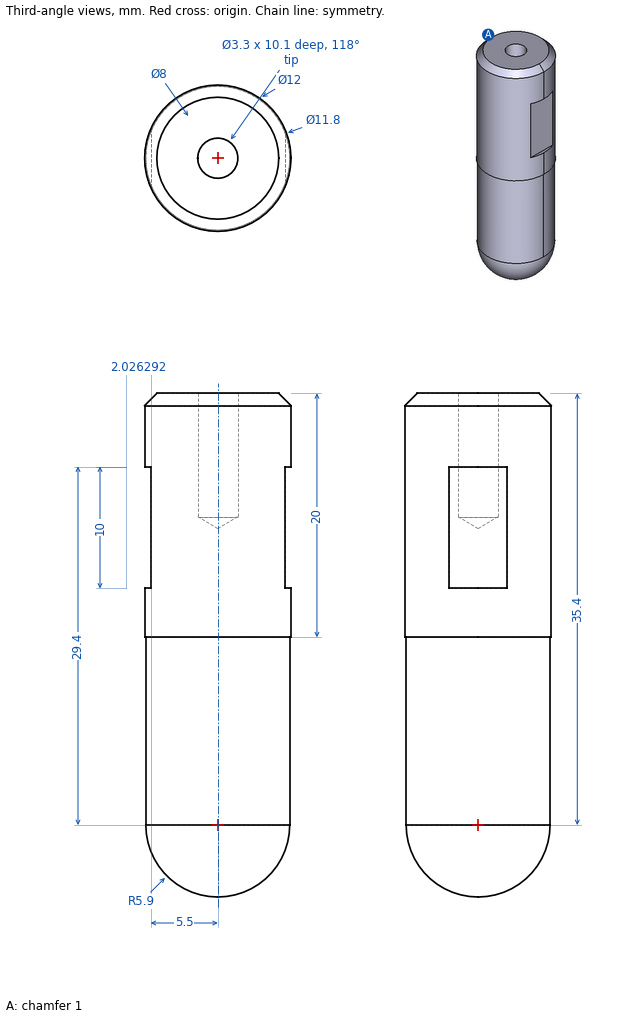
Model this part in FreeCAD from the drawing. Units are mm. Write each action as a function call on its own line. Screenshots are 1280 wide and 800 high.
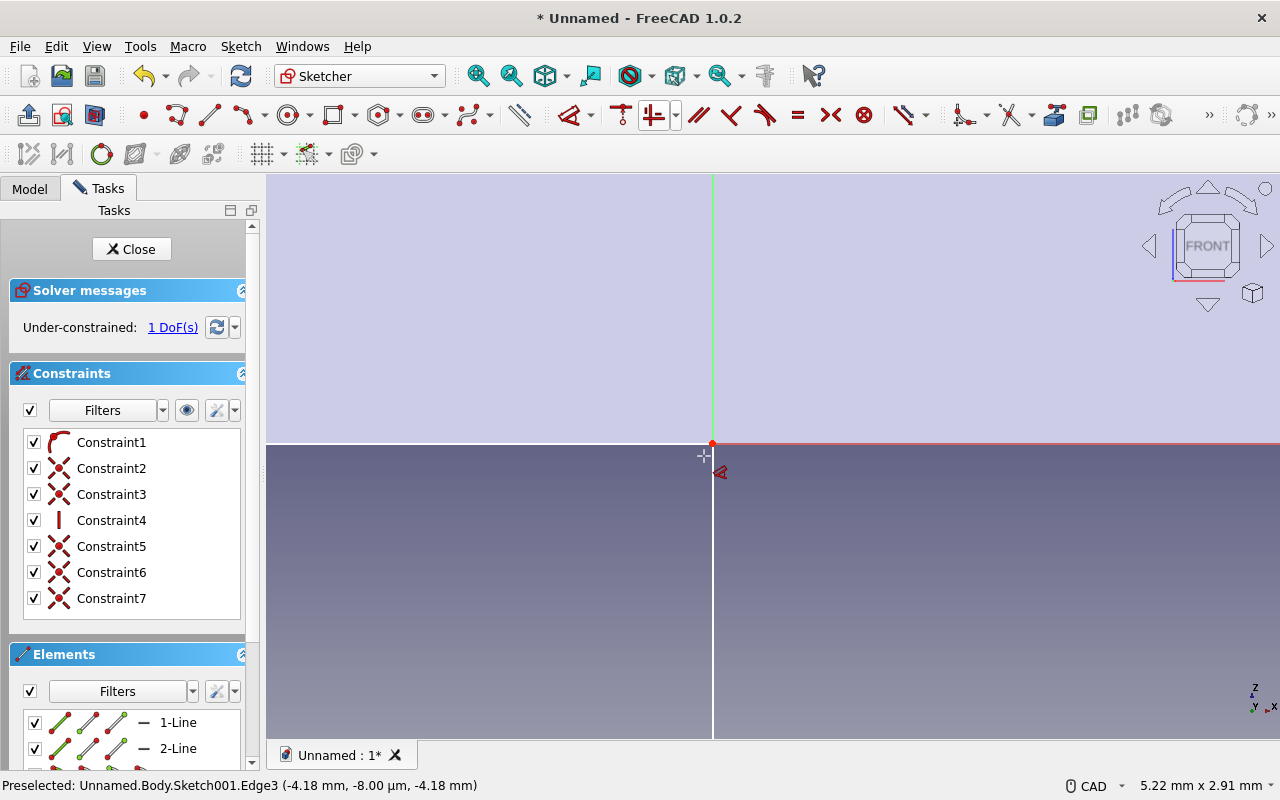
scroll(948, 215, down, 6)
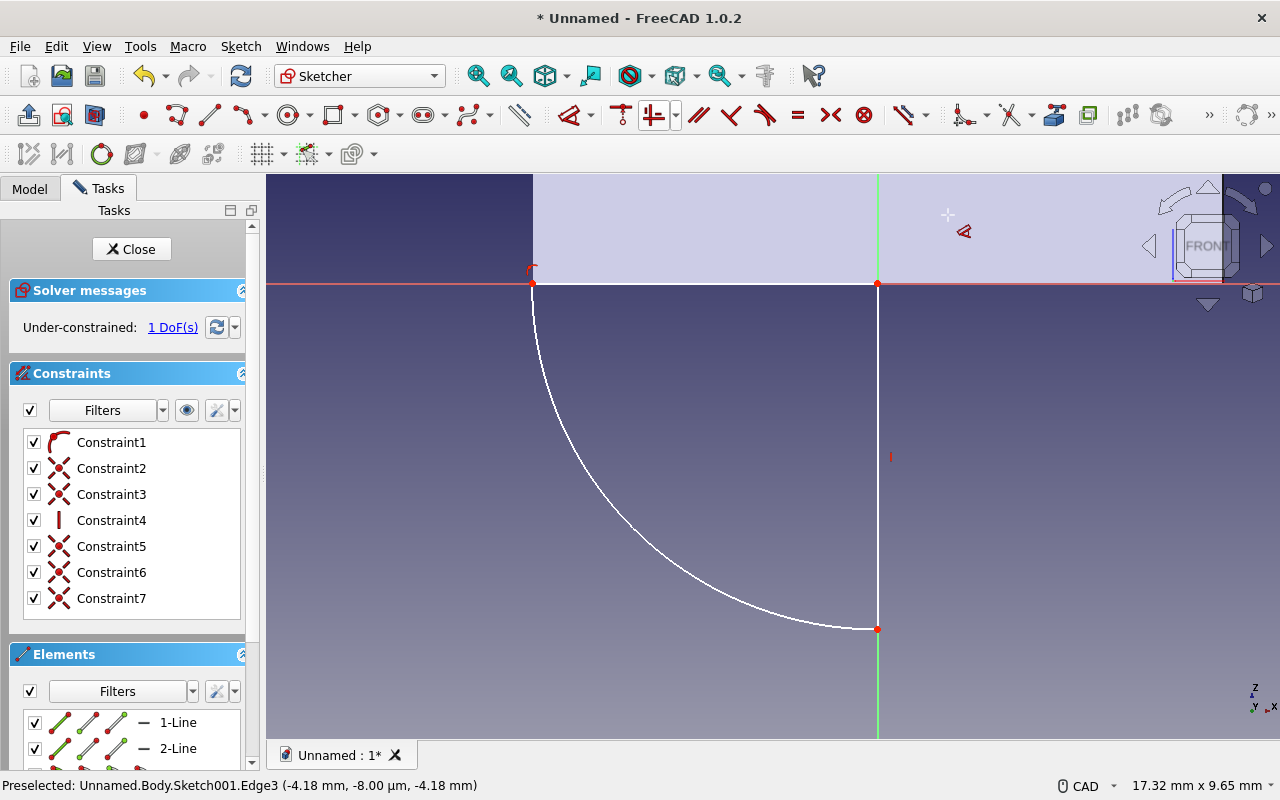
click(570, 441)
click(542, 456)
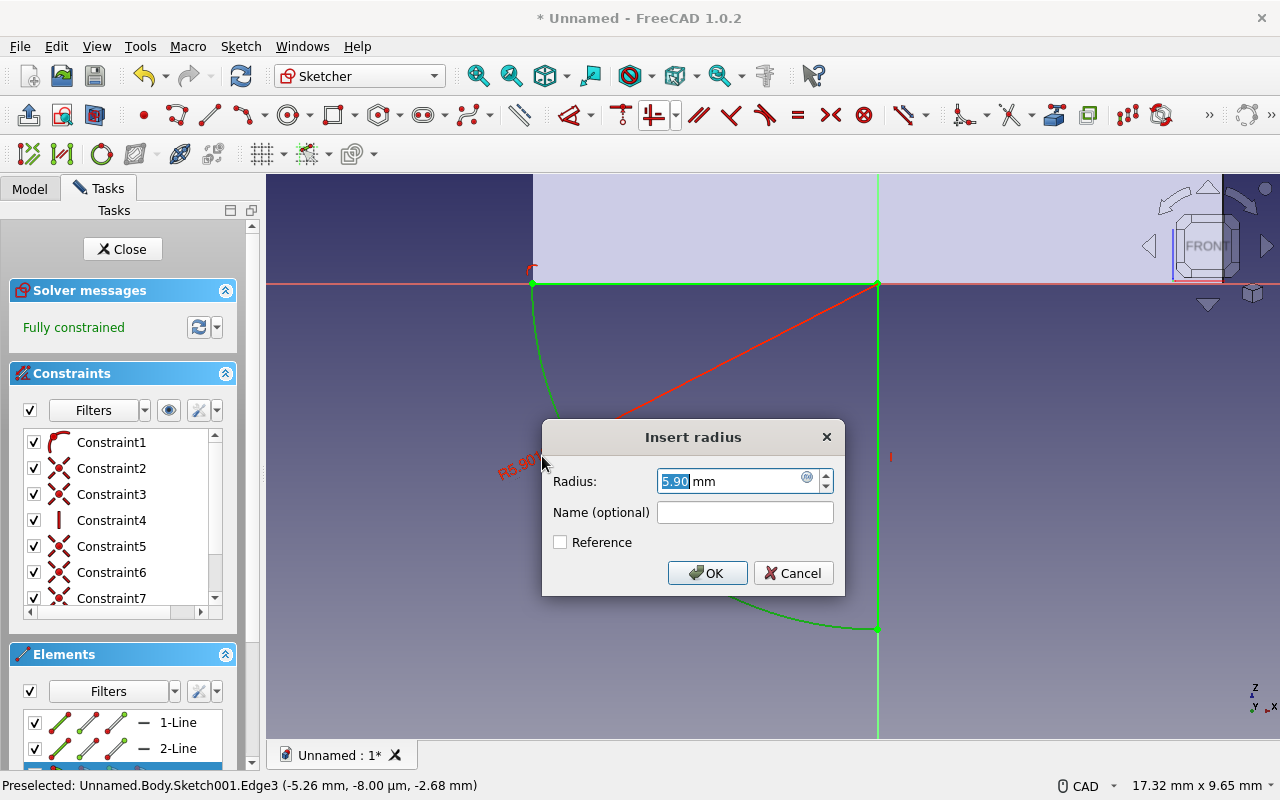
text(5.9)
key(Return)
key(Escape)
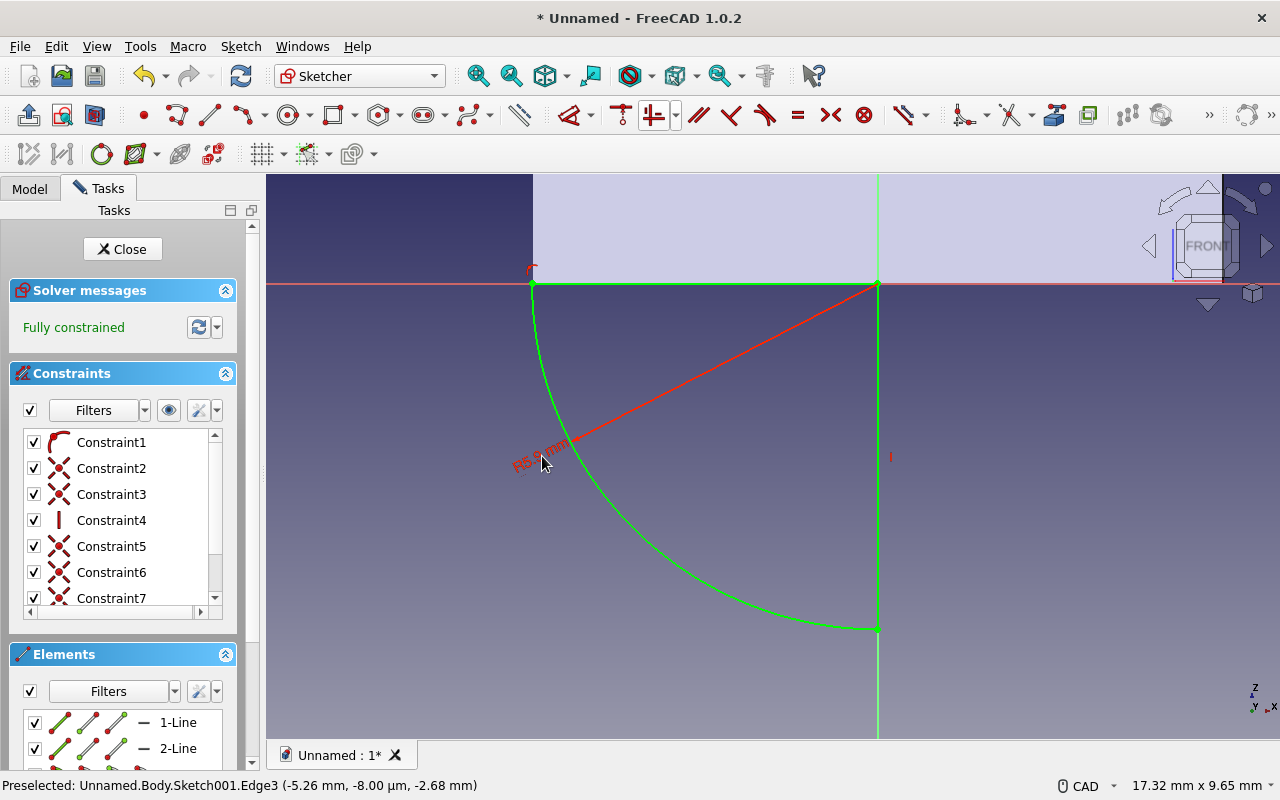
click(123, 249)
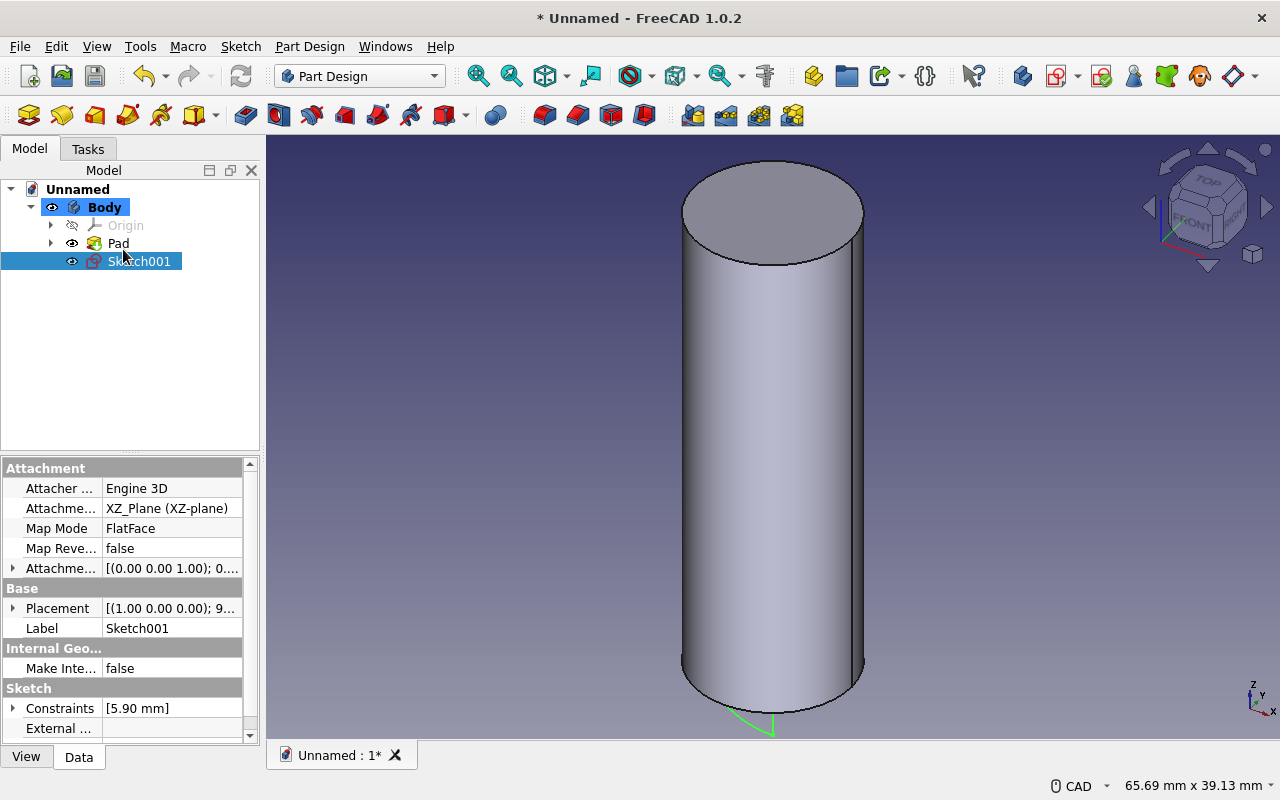
click(62, 116)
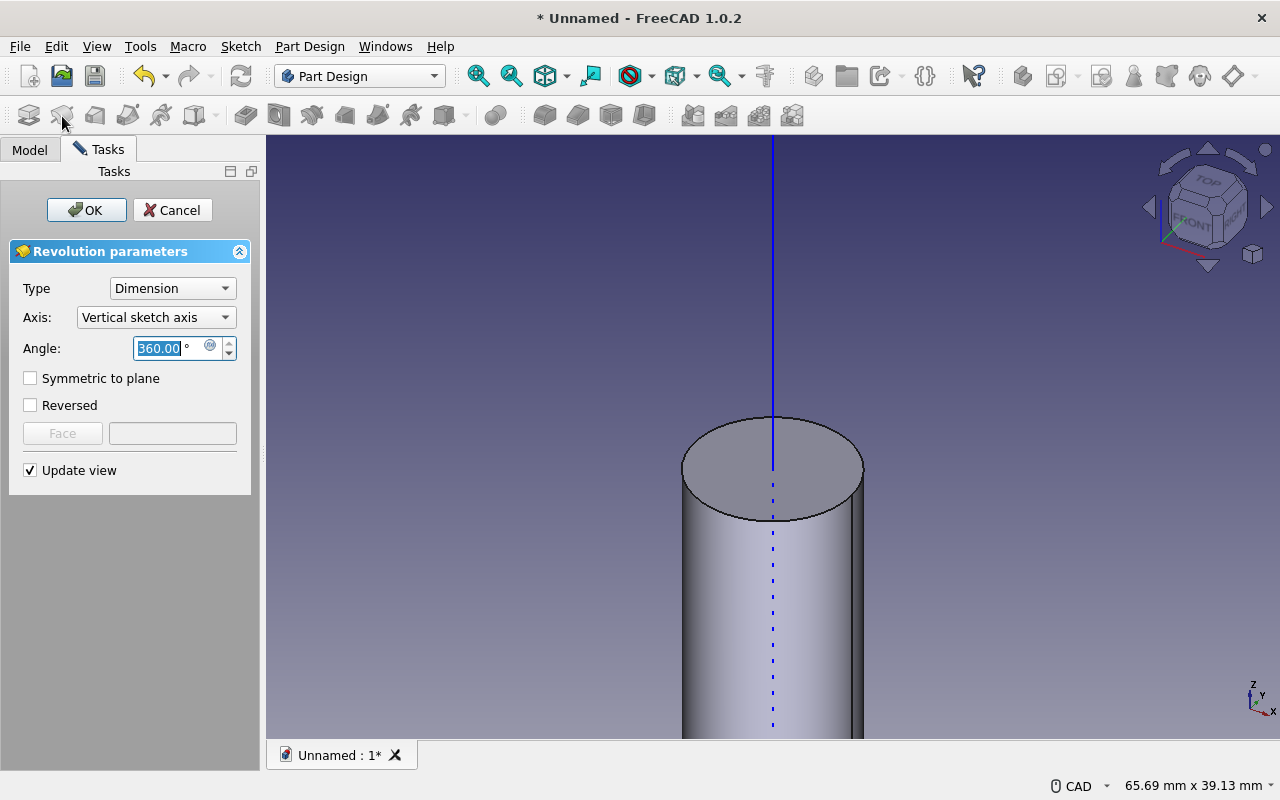
click(87, 210)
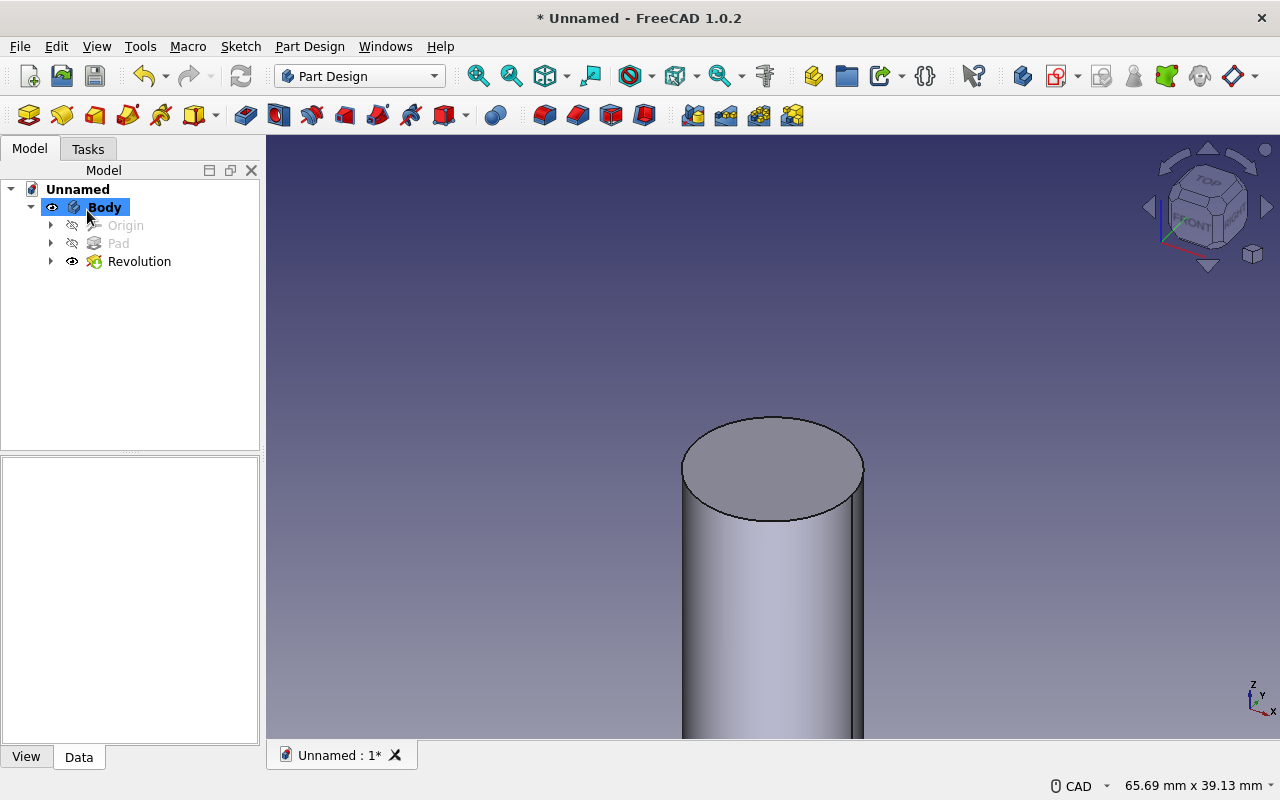
click(479, 76)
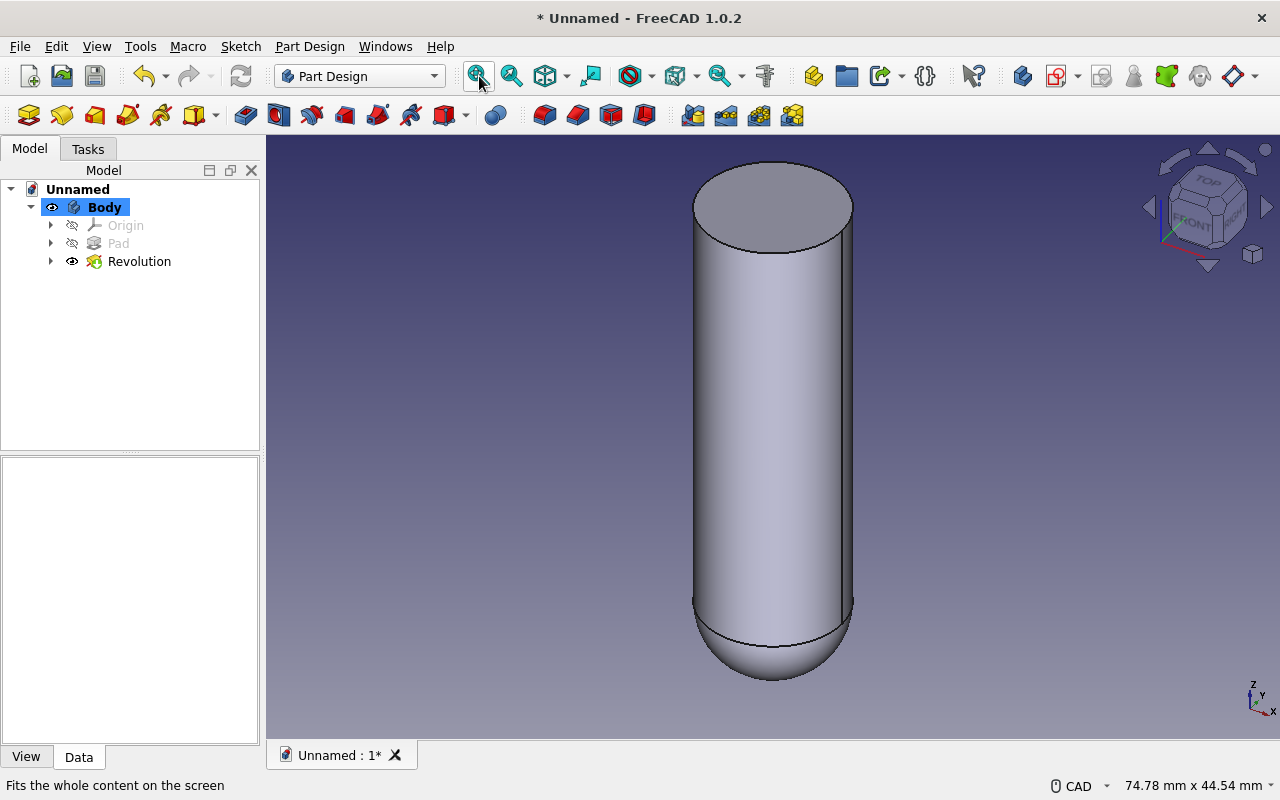
click(773, 207)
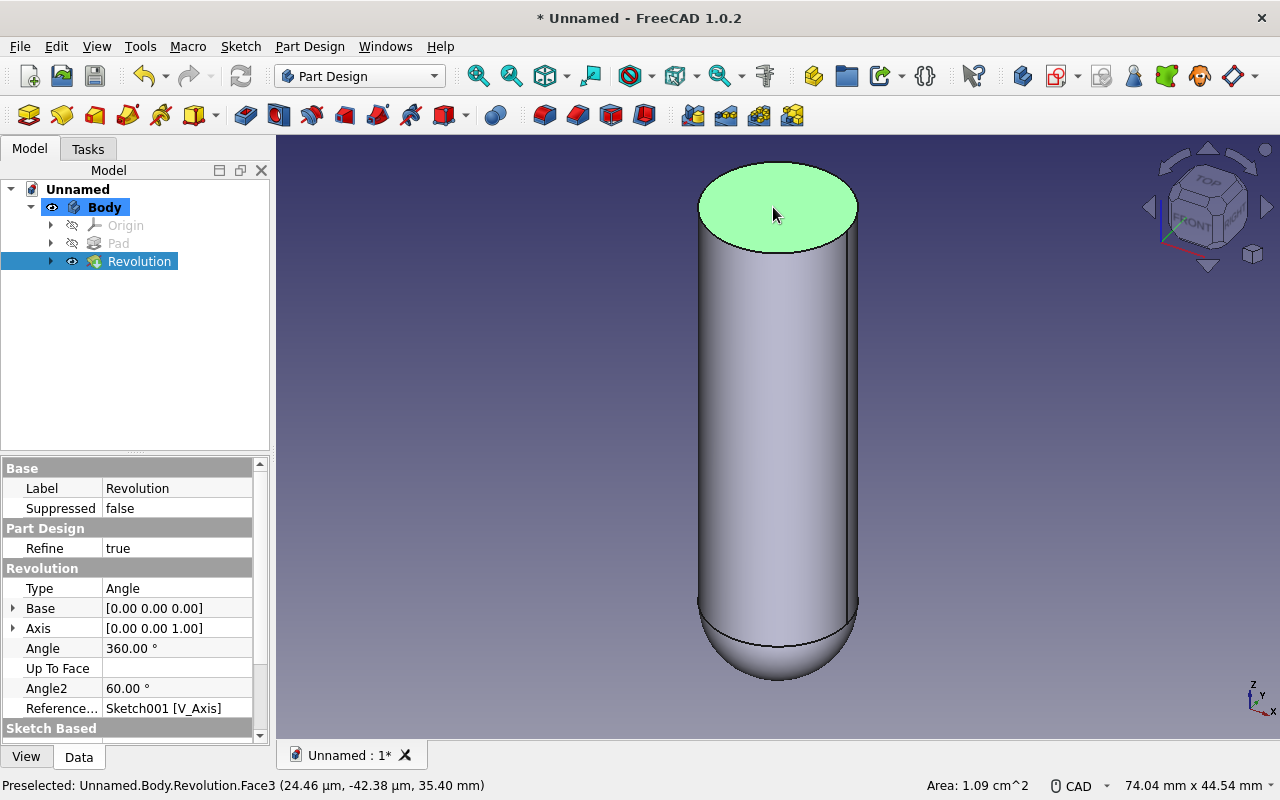
click(1056, 76)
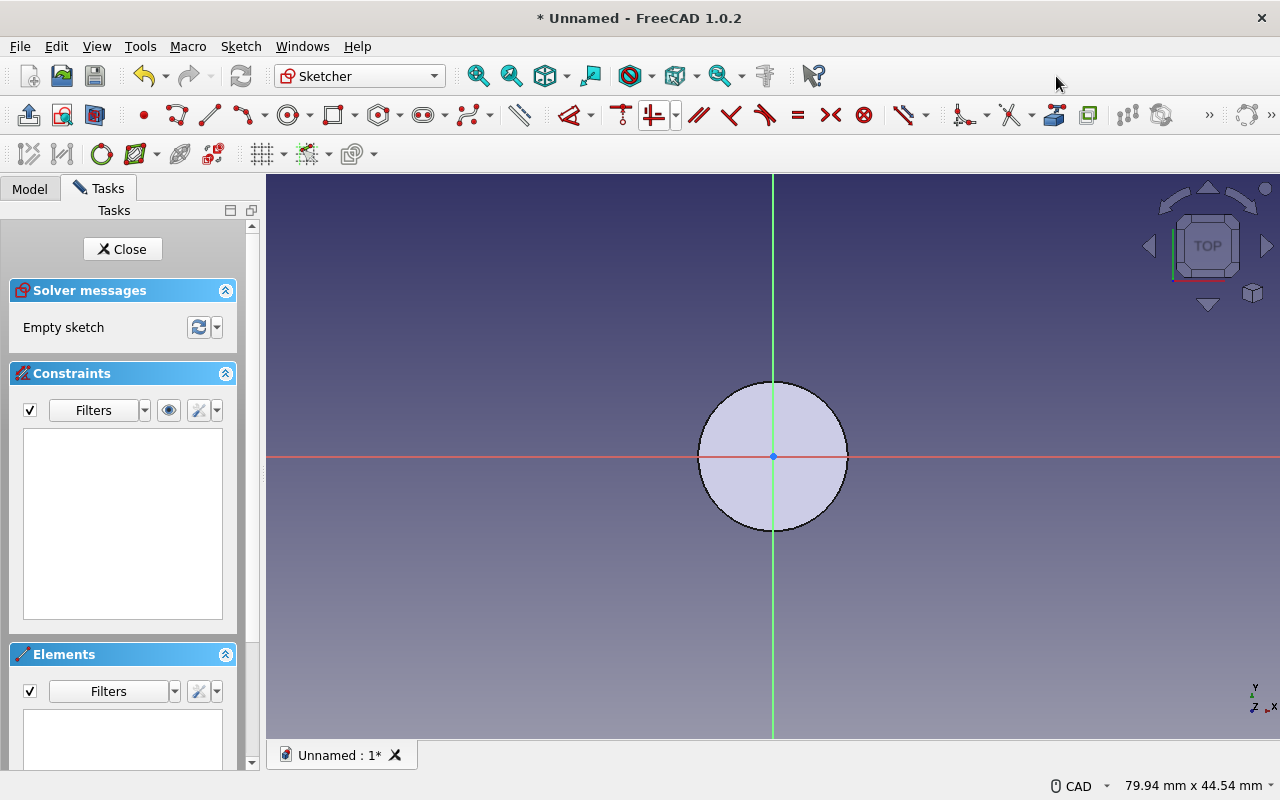
scroll(782, 456, up, 11)